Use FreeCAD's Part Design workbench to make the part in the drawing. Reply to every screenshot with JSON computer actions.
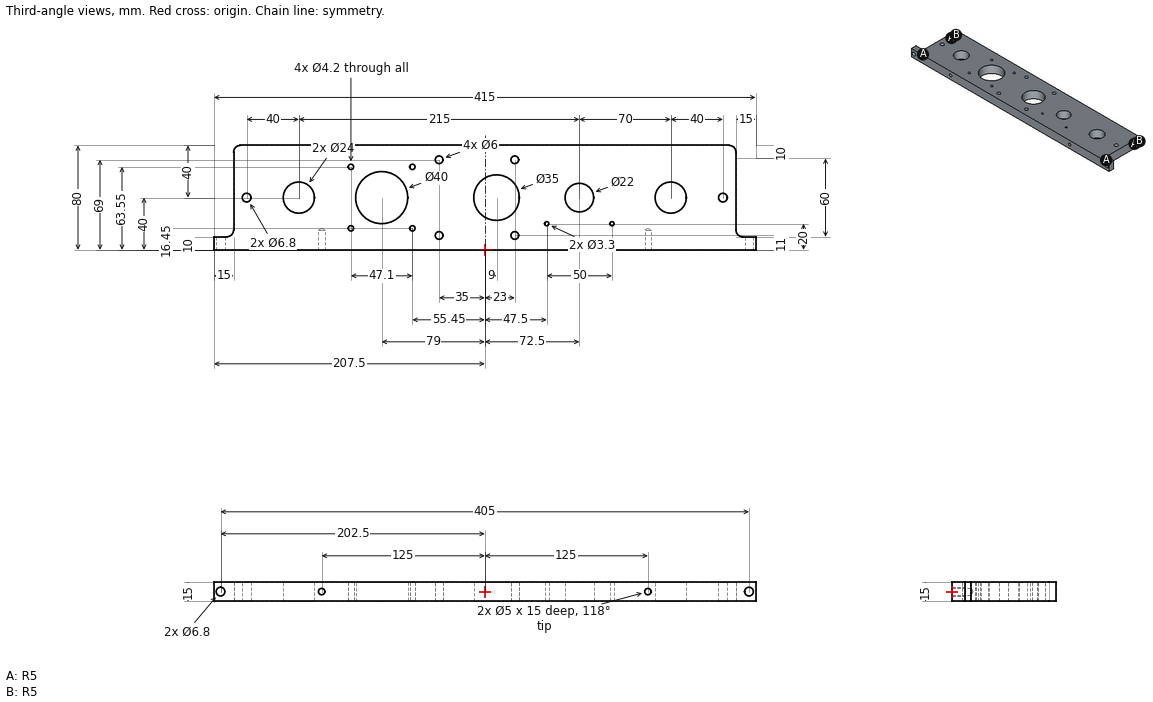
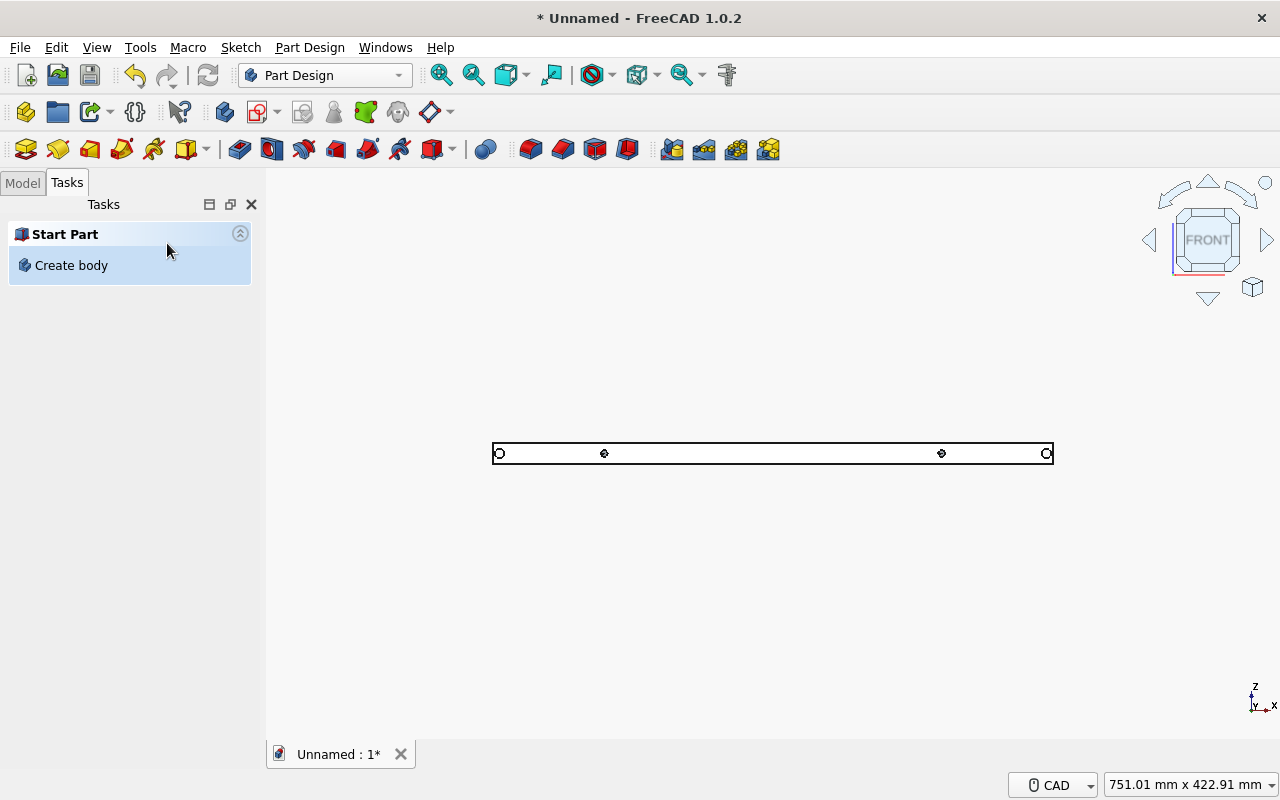
{"action": "key", "text": "0"}